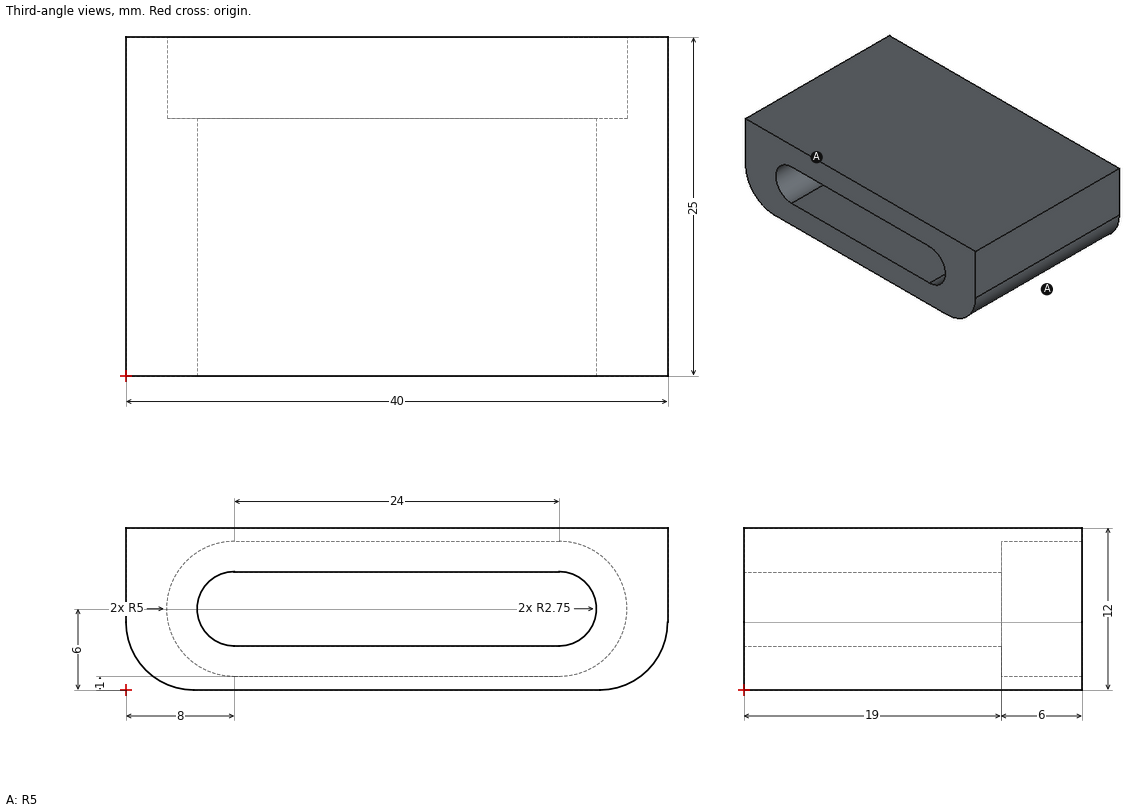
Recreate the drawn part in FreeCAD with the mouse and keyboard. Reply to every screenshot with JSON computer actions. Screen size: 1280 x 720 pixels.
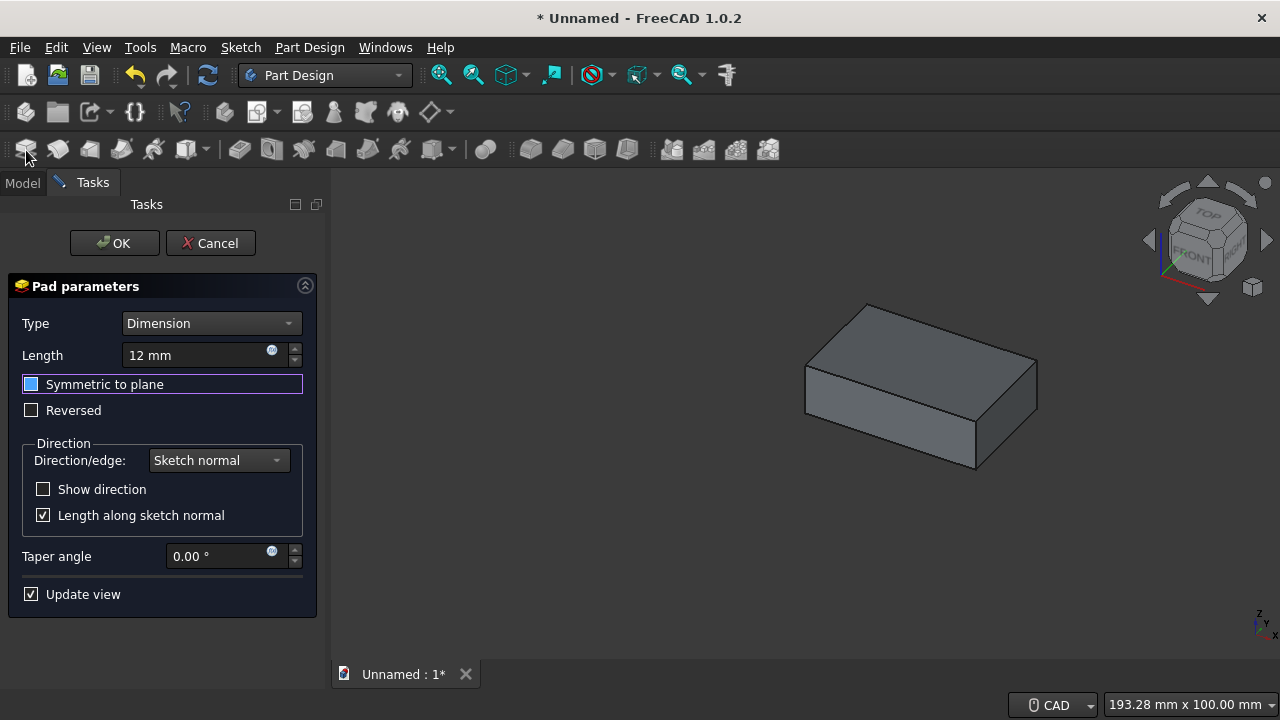
{"action": "left_click", "coordinate": [115, 243]}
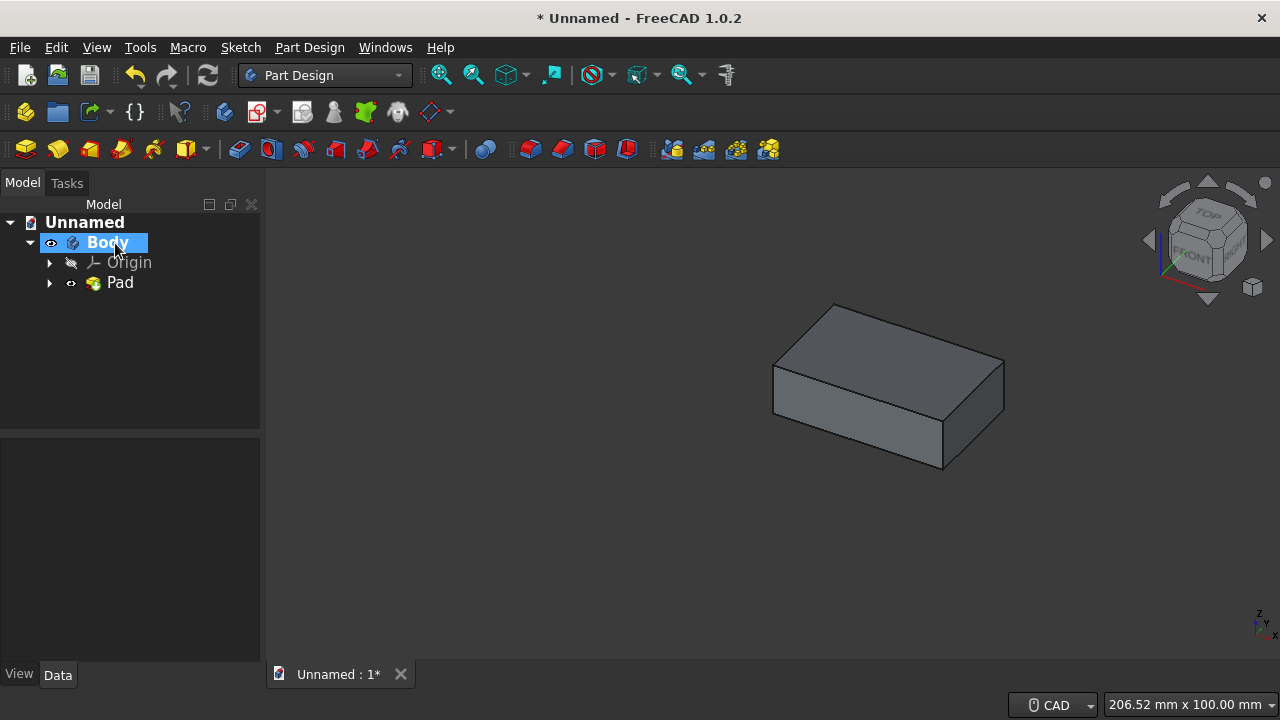
{"action": "key", "text": "v f"}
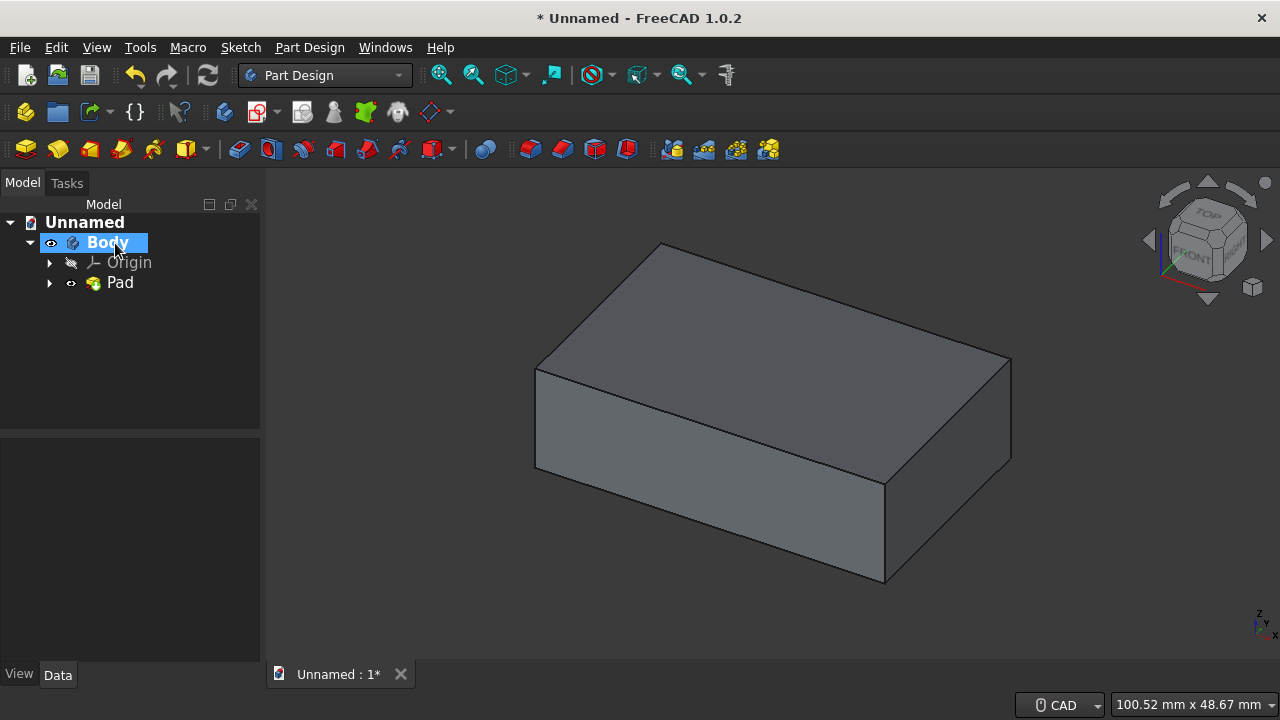
{"action": "key", "text": "4"}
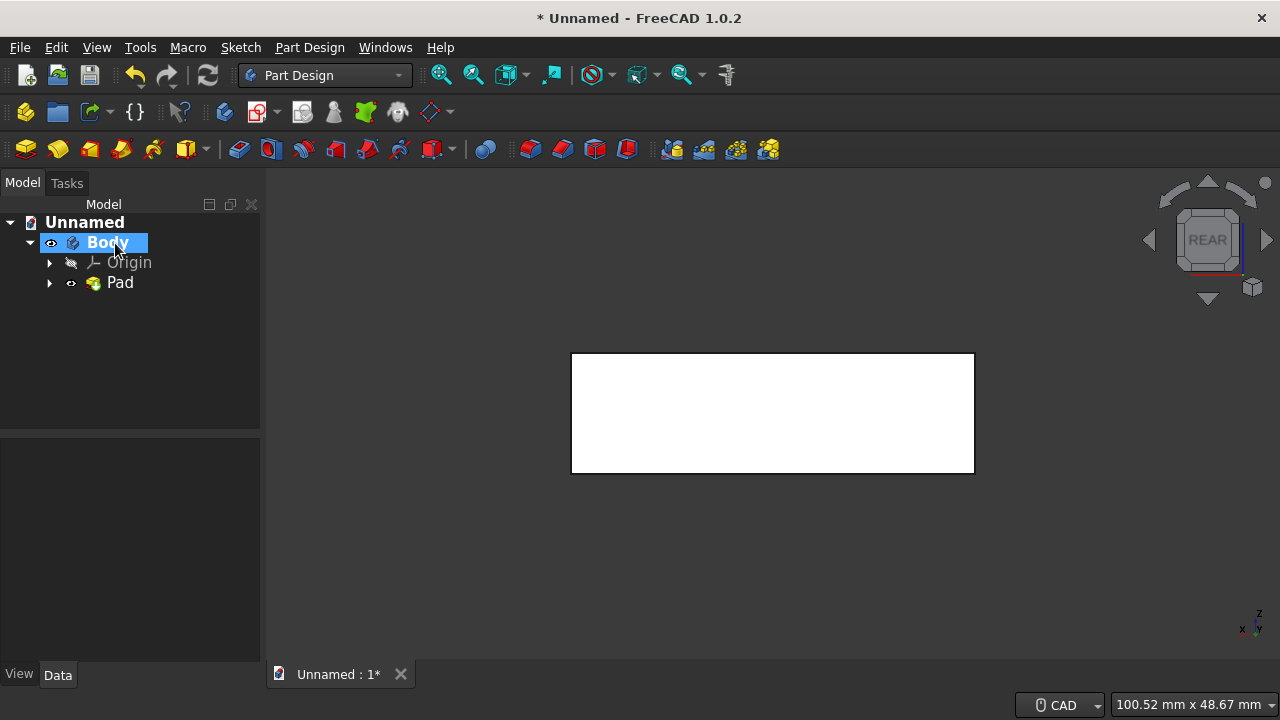
{"action": "left_click", "coordinate": [442, 76]}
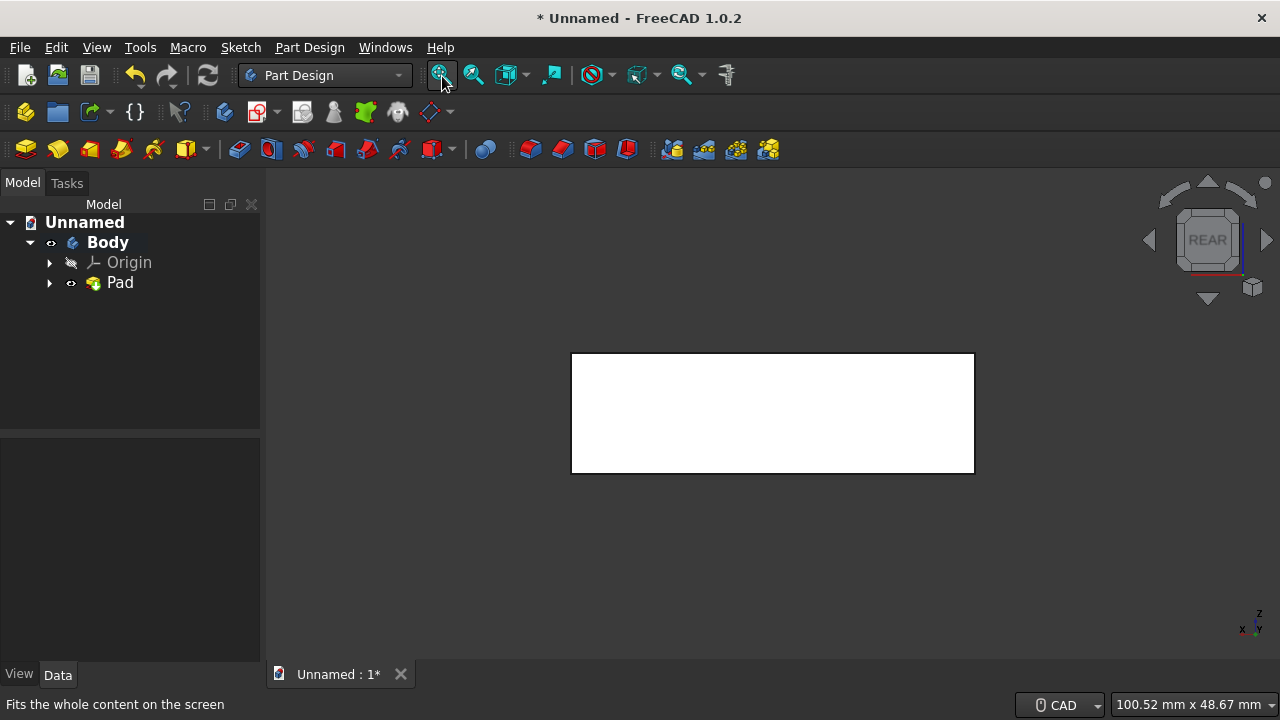
{"action": "left_click", "coordinate": [658, 413]}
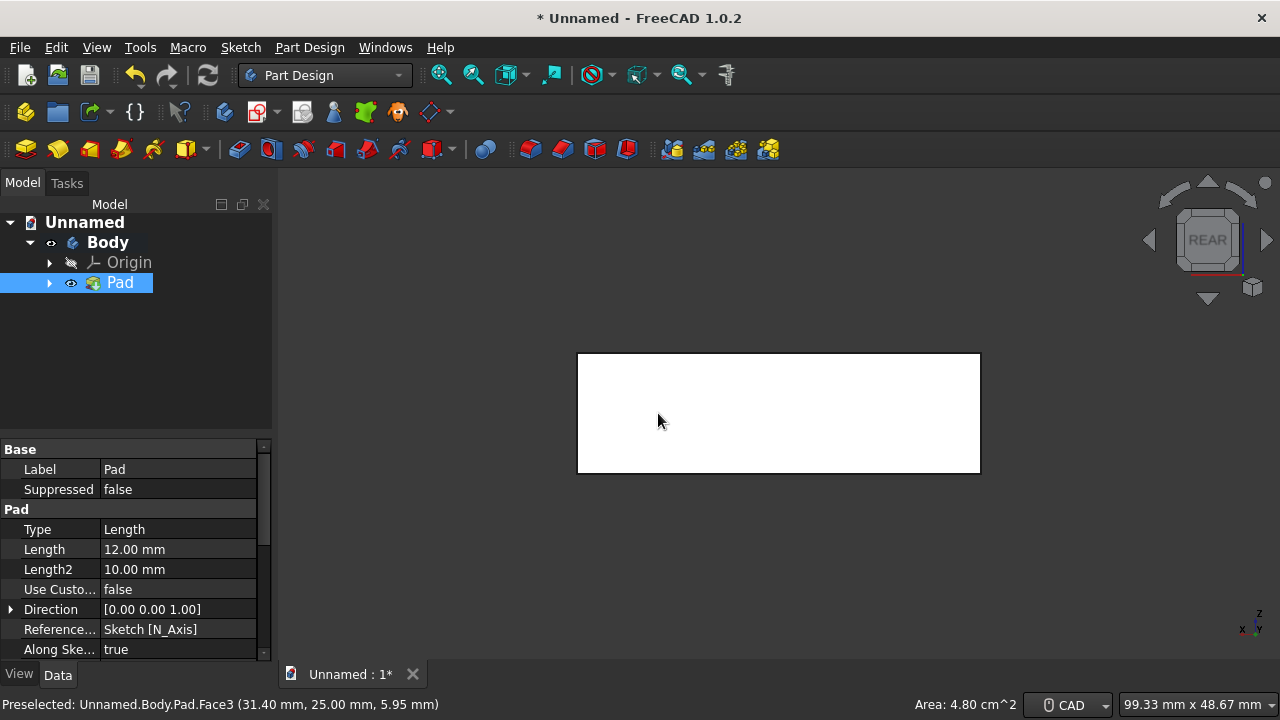
{"action": "left_click", "coordinate": [258, 112]}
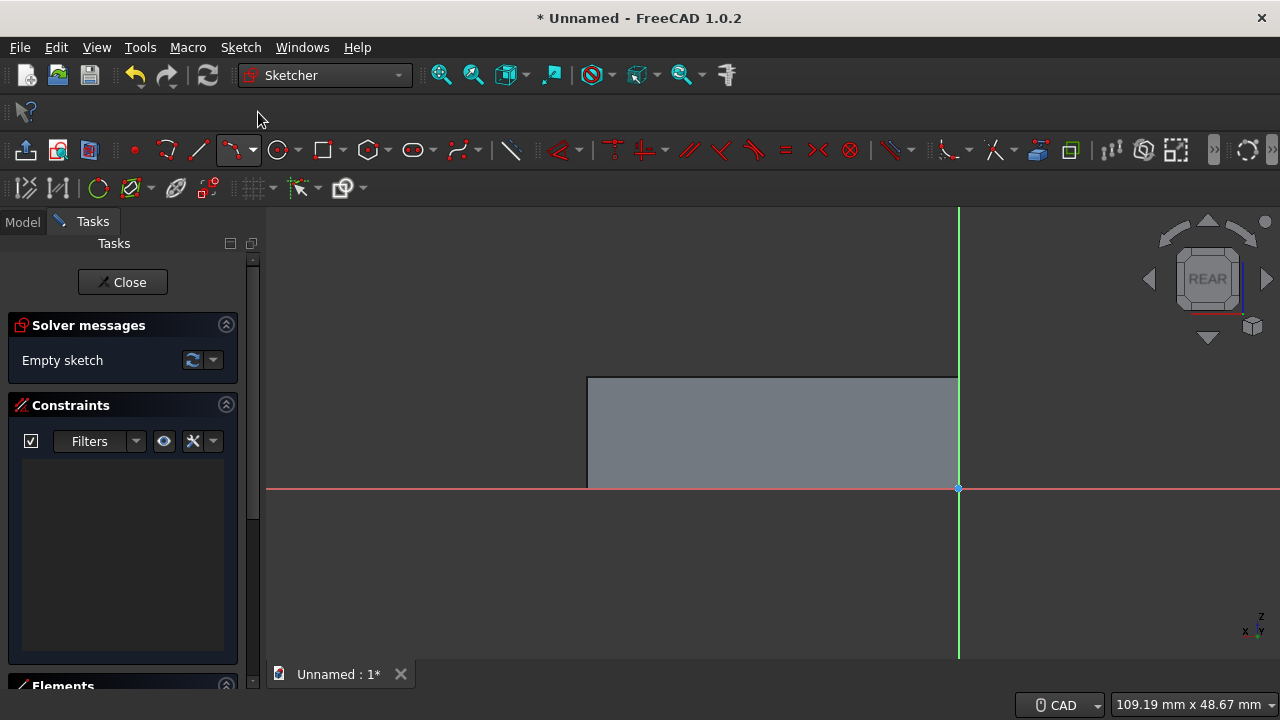
{"action": "scroll", "coordinate": [887, 443], "scroll_direction": "up", "scroll_amount": 3}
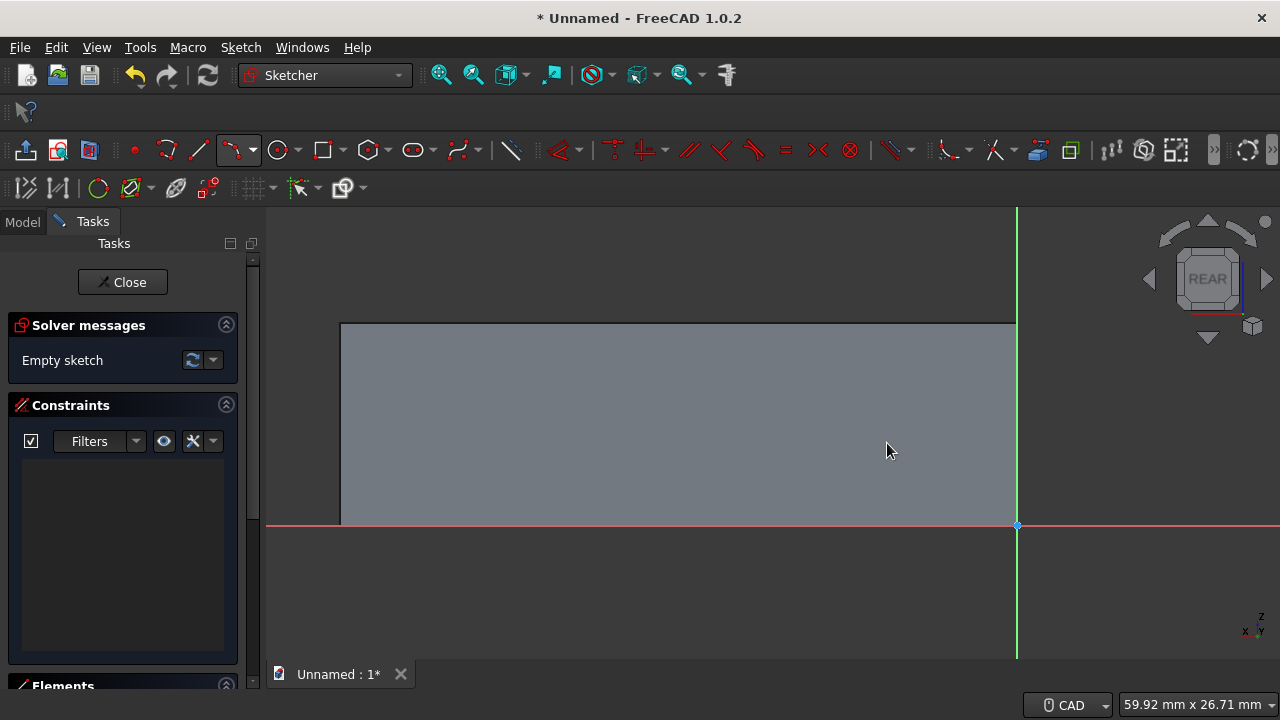
{"action": "key", "text": "g s"}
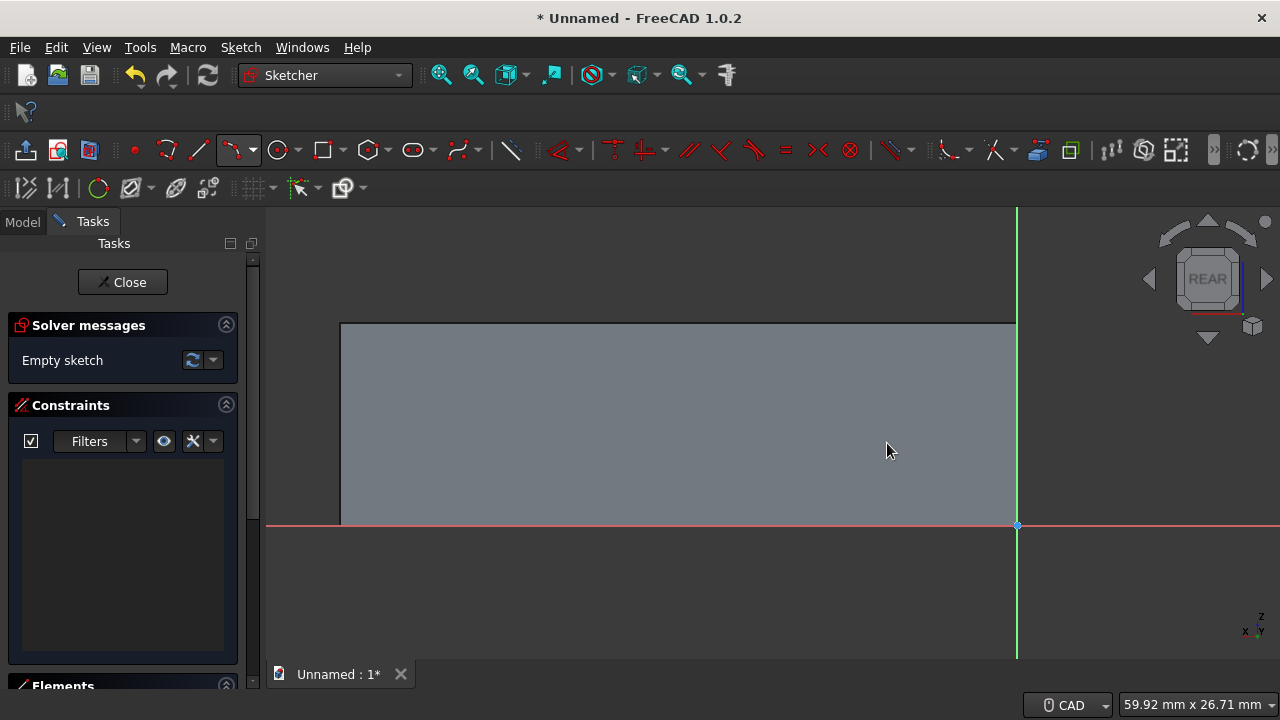
{"action": "left_click", "coordinate": [476, 424]}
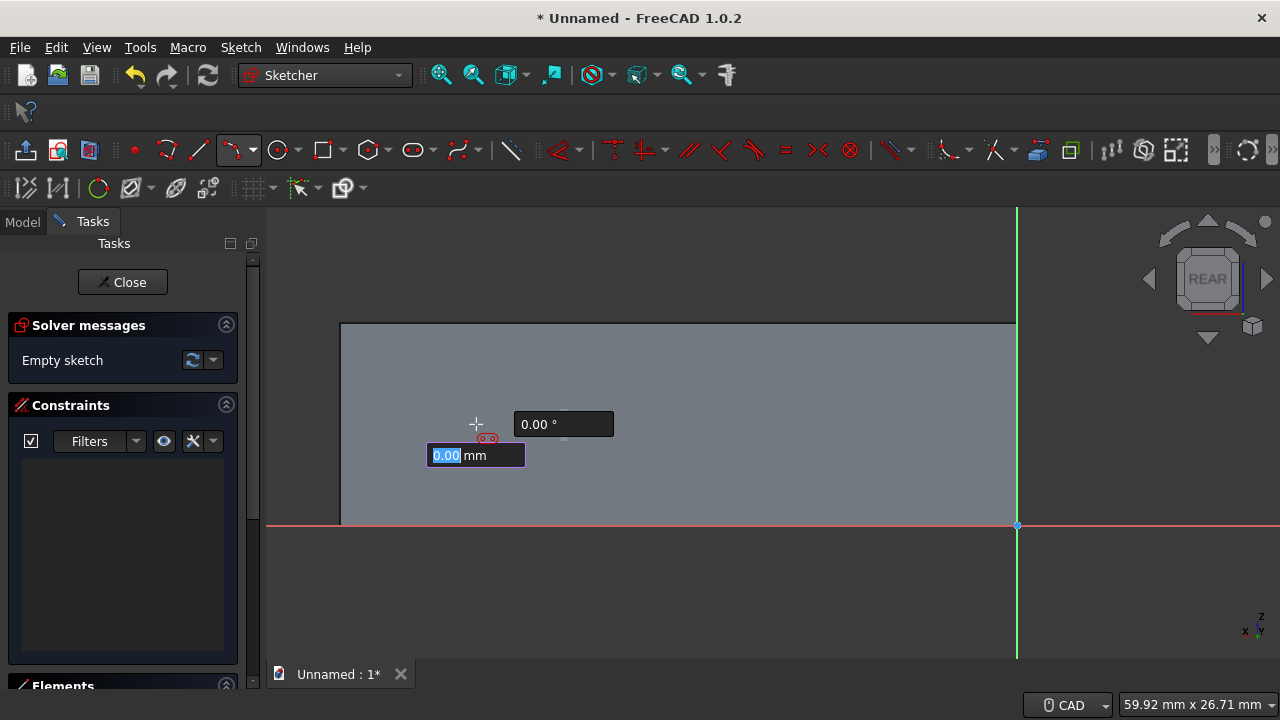
{"action": "left_click", "coordinate": [882, 424]}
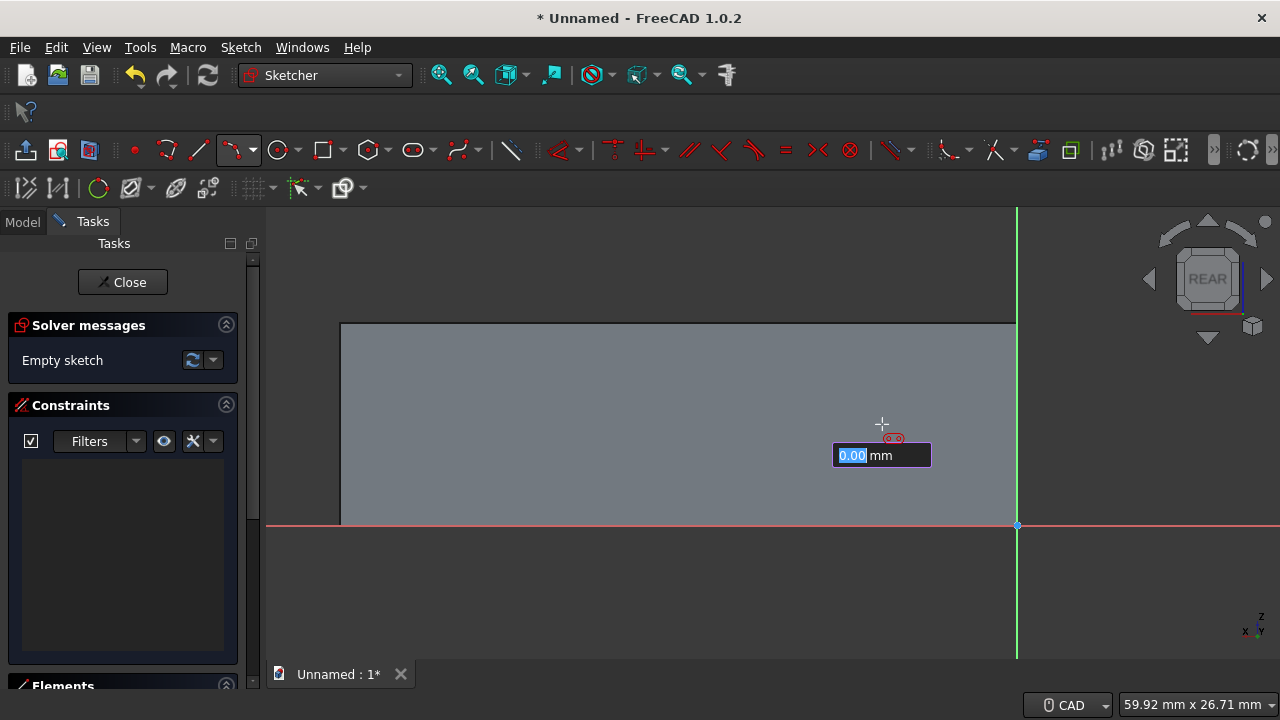
{"action": "left_click", "coordinate": [679, 509]}
{"action": "key", "text": "Escape"}